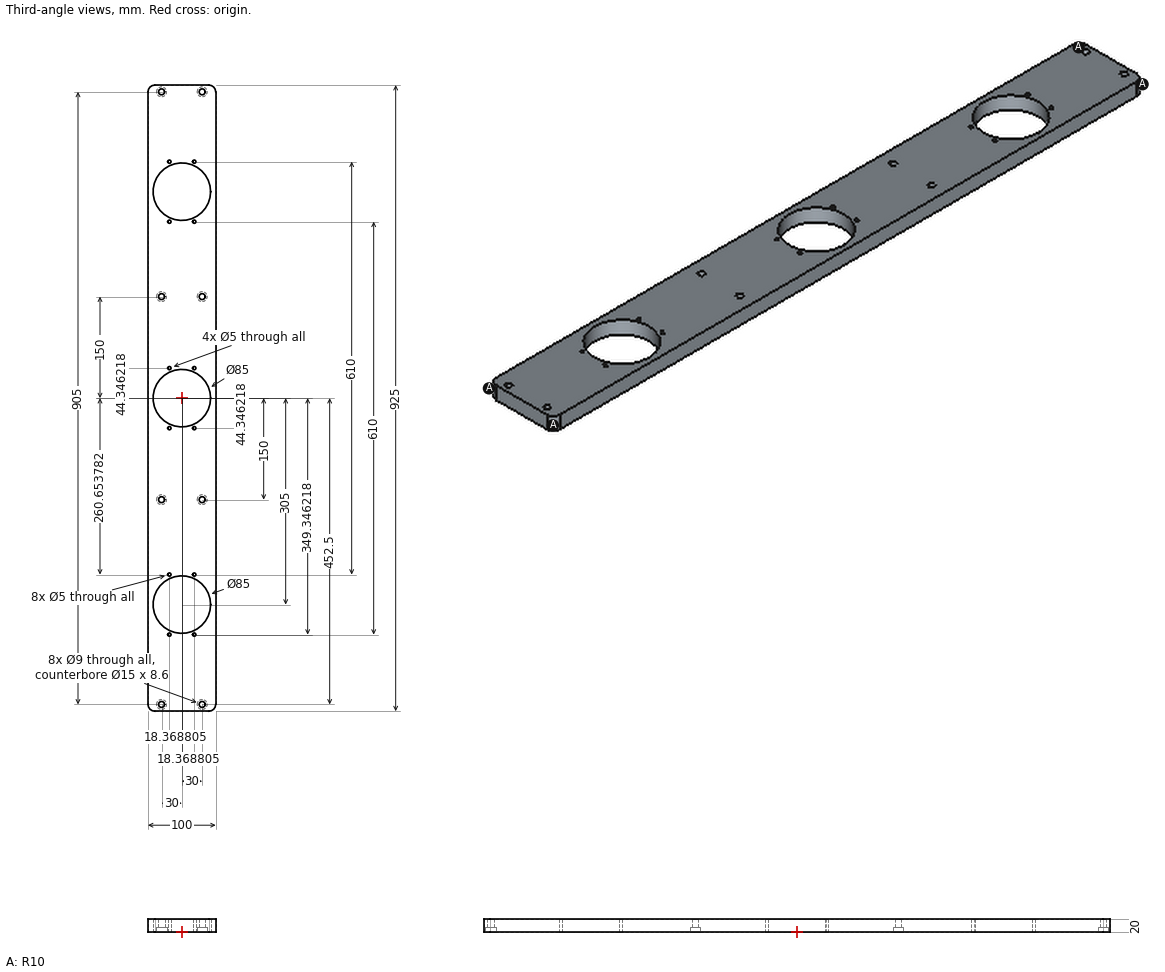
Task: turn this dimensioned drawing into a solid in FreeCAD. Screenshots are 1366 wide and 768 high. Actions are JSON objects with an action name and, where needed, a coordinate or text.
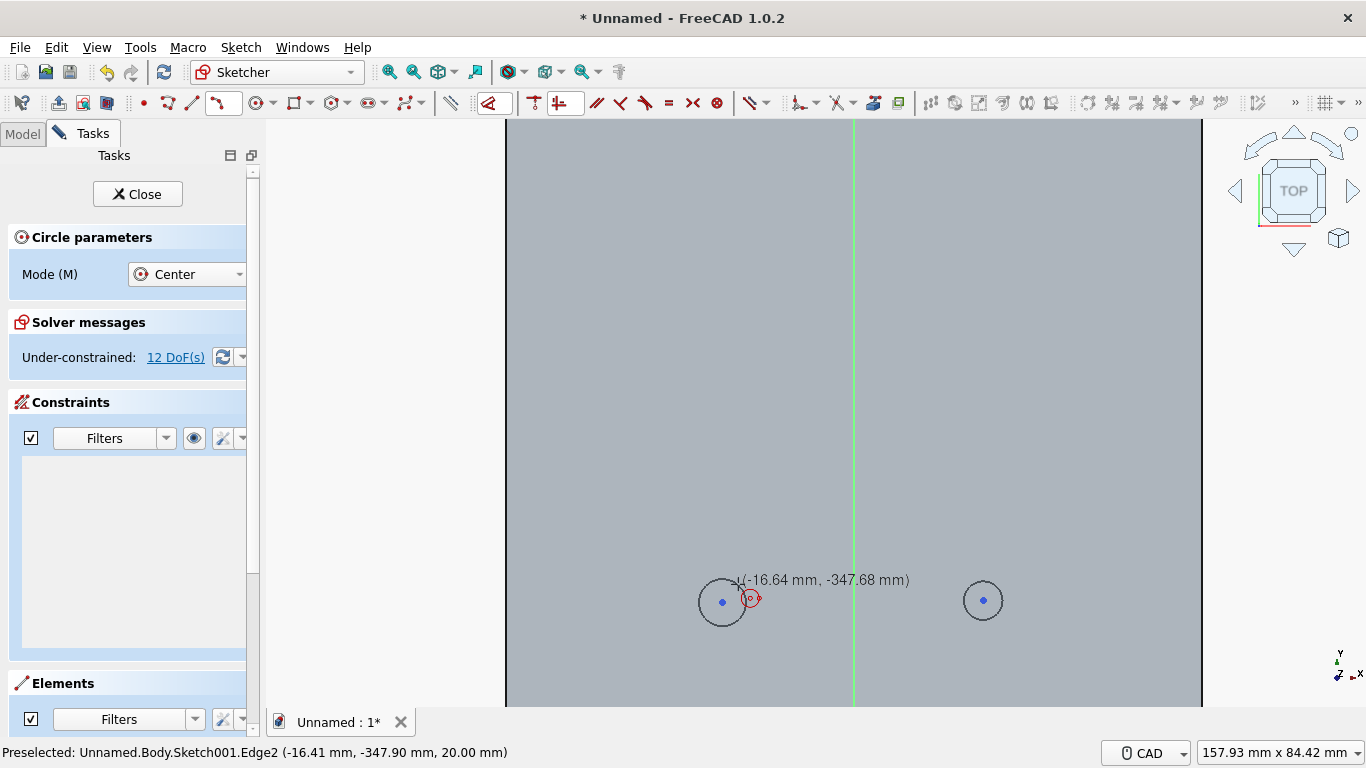
{"action": "scroll", "coordinate": [739, 593], "scroll_direction": "down", "scroll_amount": 13}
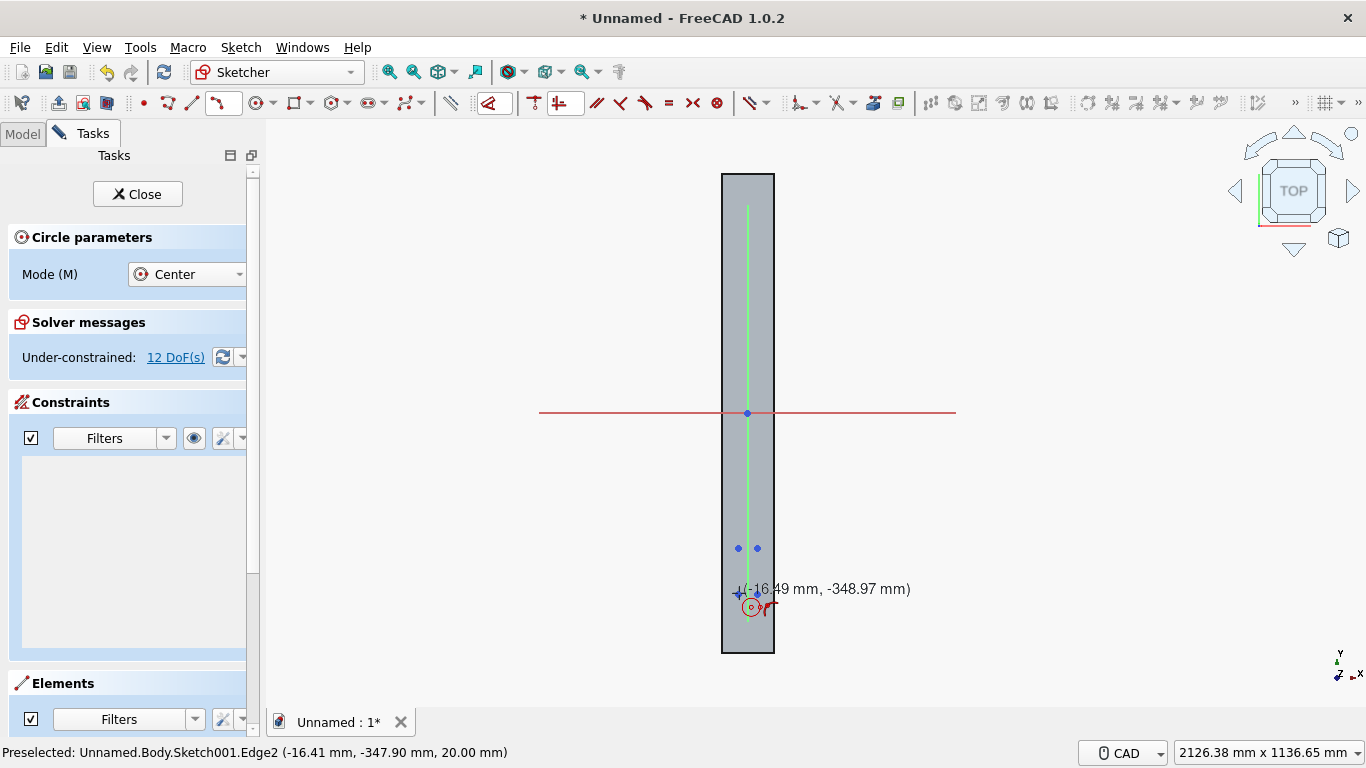
{"action": "scroll", "coordinate": [757, 233], "scroll_direction": "up", "scroll_amount": 15}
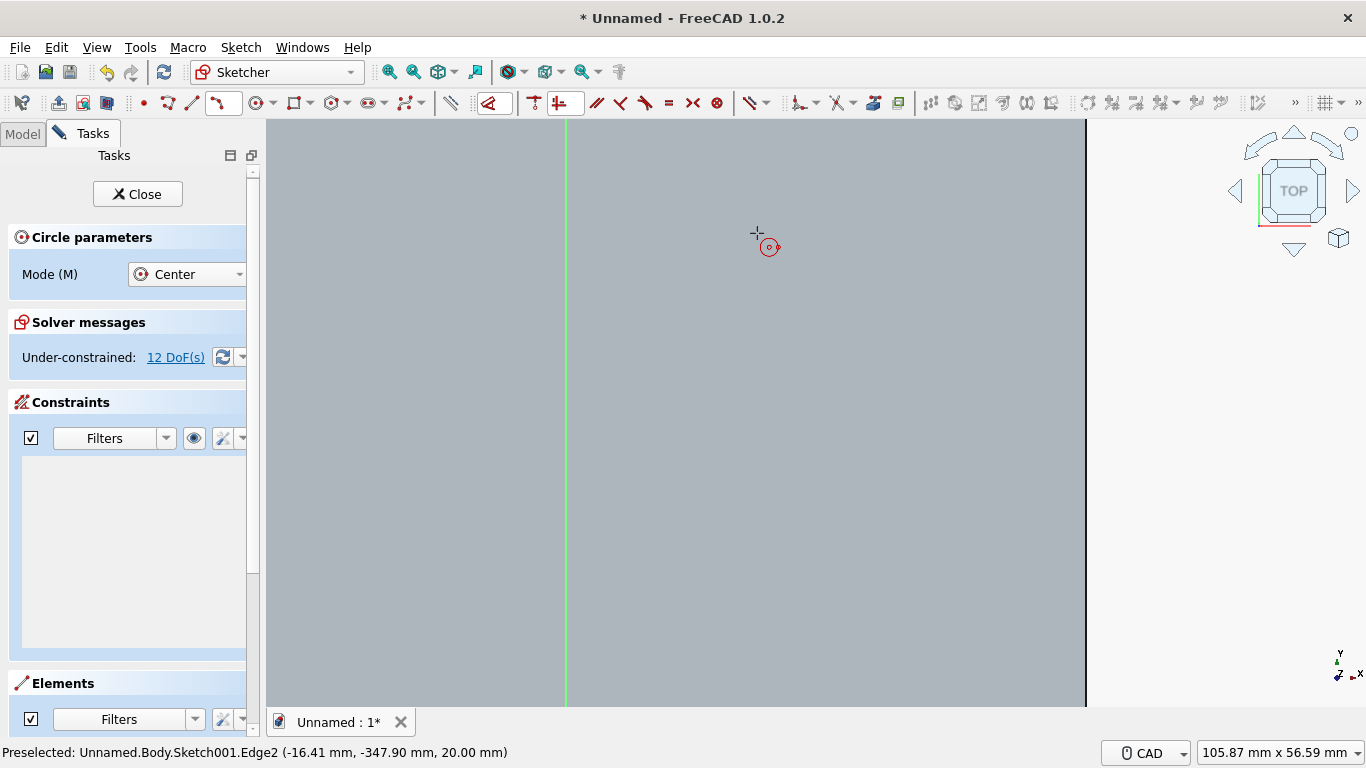
{"action": "scroll", "coordinate": [757, 233], "scroll_direction": "down", "scroll_amount": 15}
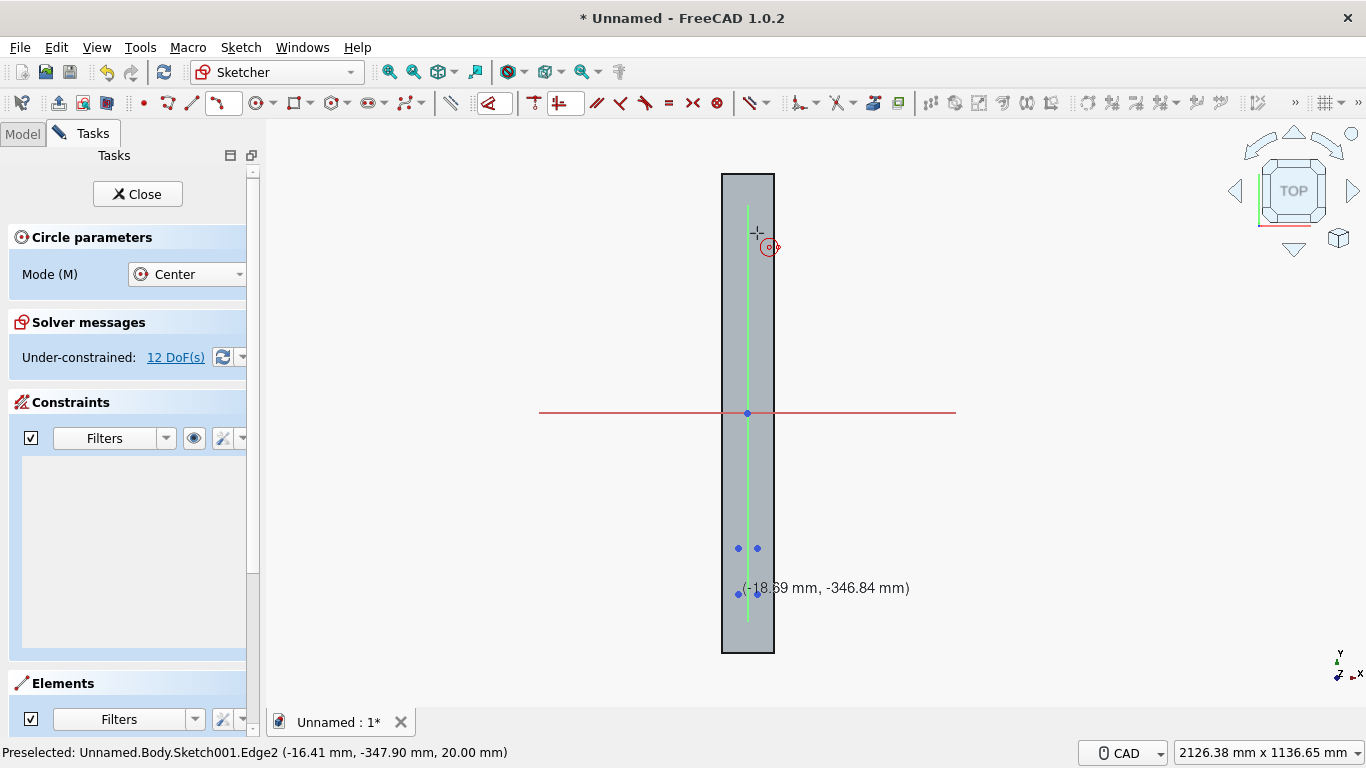
{"action": "scroll", "coordinate": [757, 233], "scroll_direction": "up", "scroll_amount": 3}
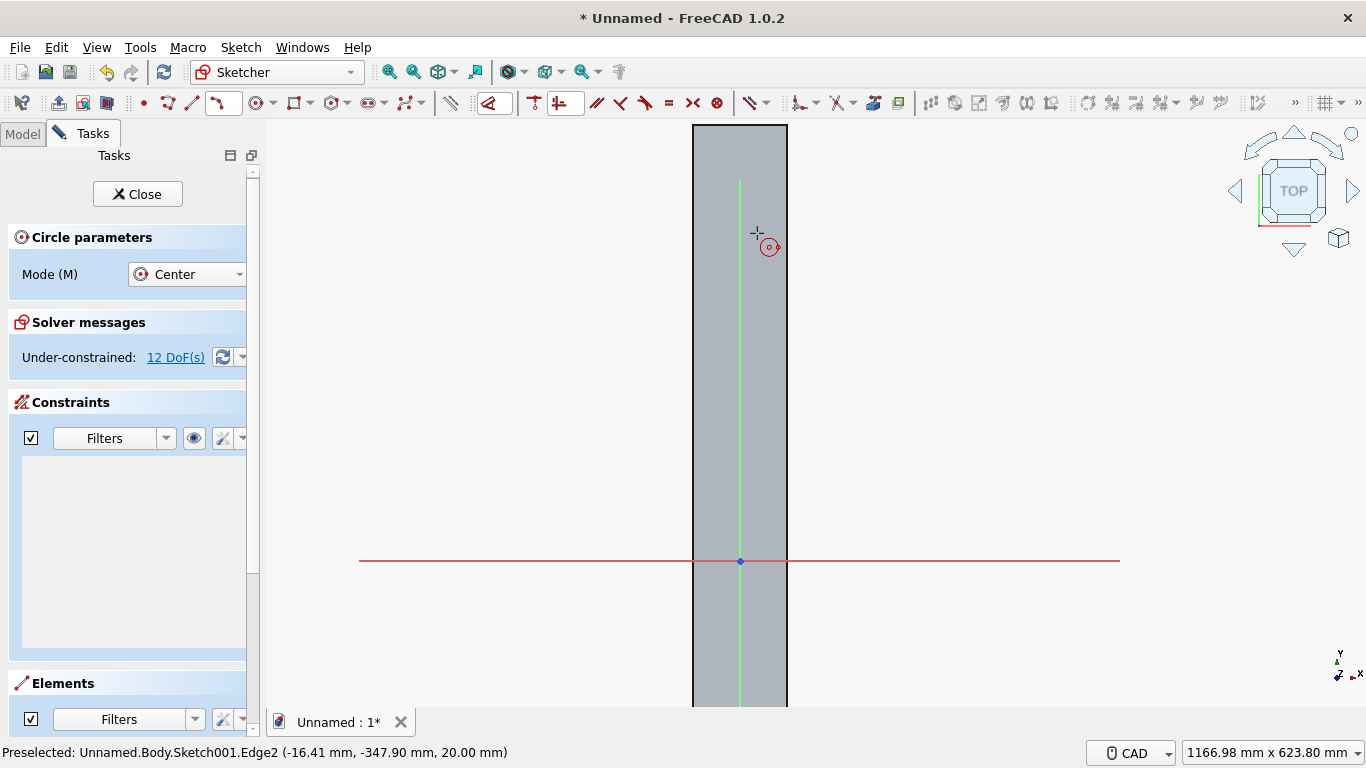
{"action": "left_click", "coordinate": [757, 232]}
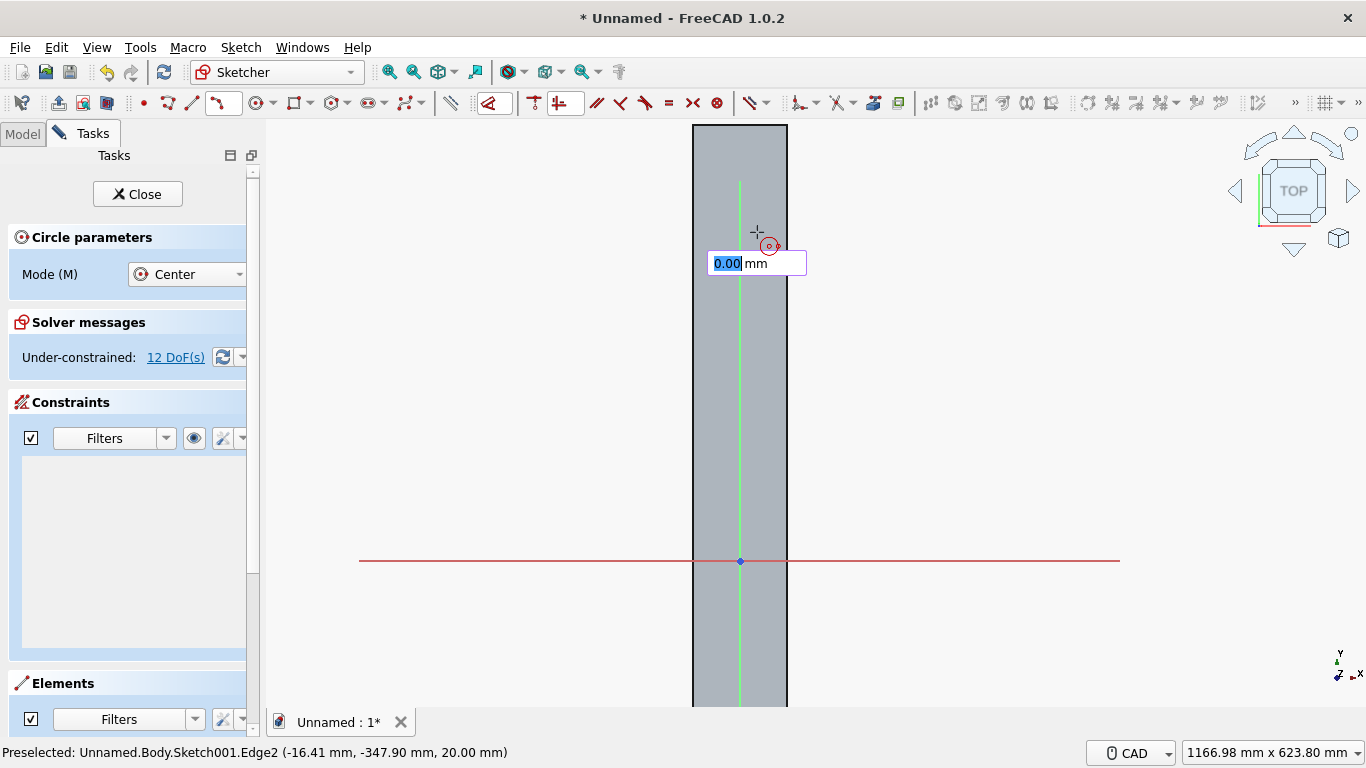
{"action": "scroll", "coordinate": [759, 230], "scroll_direction": "up", "scroll_amount": 10}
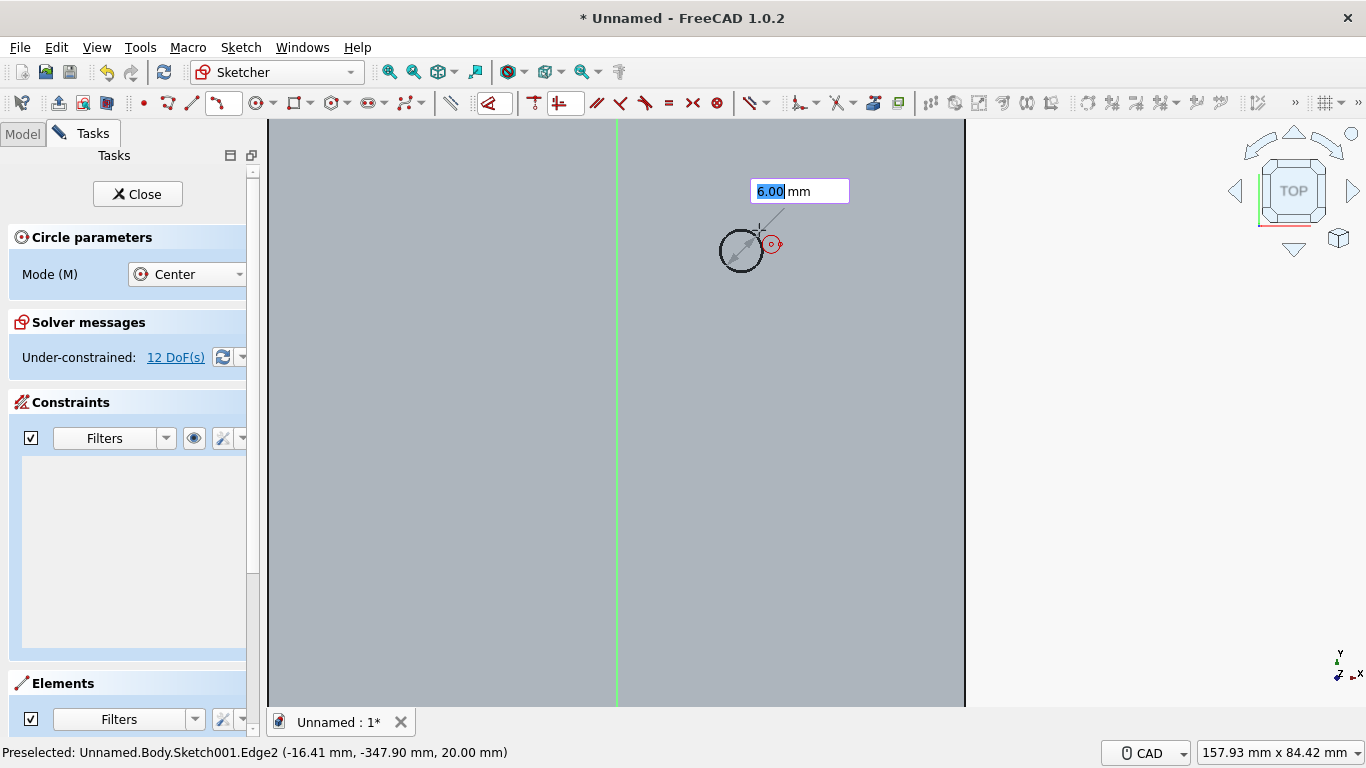
{"action": "left_click", "coordinate": [757, 232]}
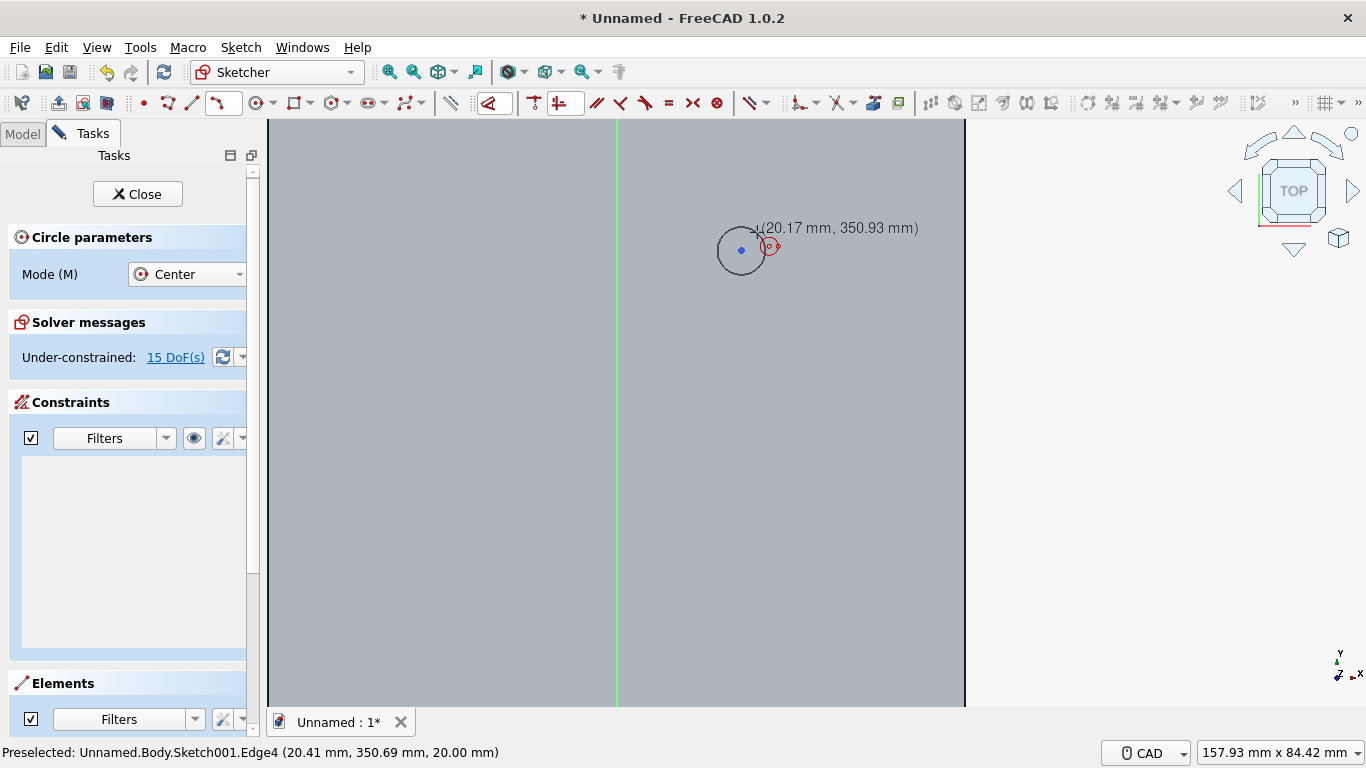
{"action": "scroll", "coordinate": [489, 244], "scroll_direction": "up", "scroll_amount": 2}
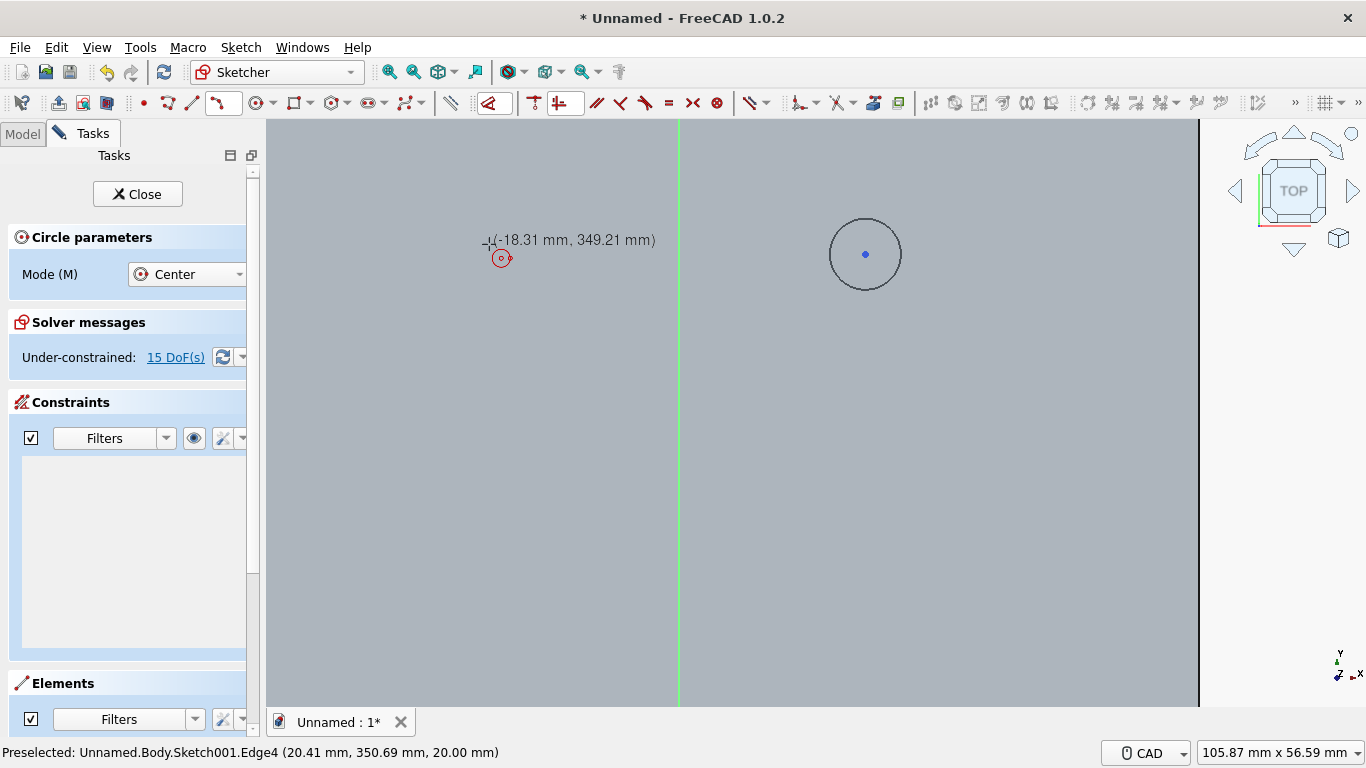
{"action": "scroll", "coordinate": [751, 232], "scroll_direction": "down", "scroll_amount": 15}